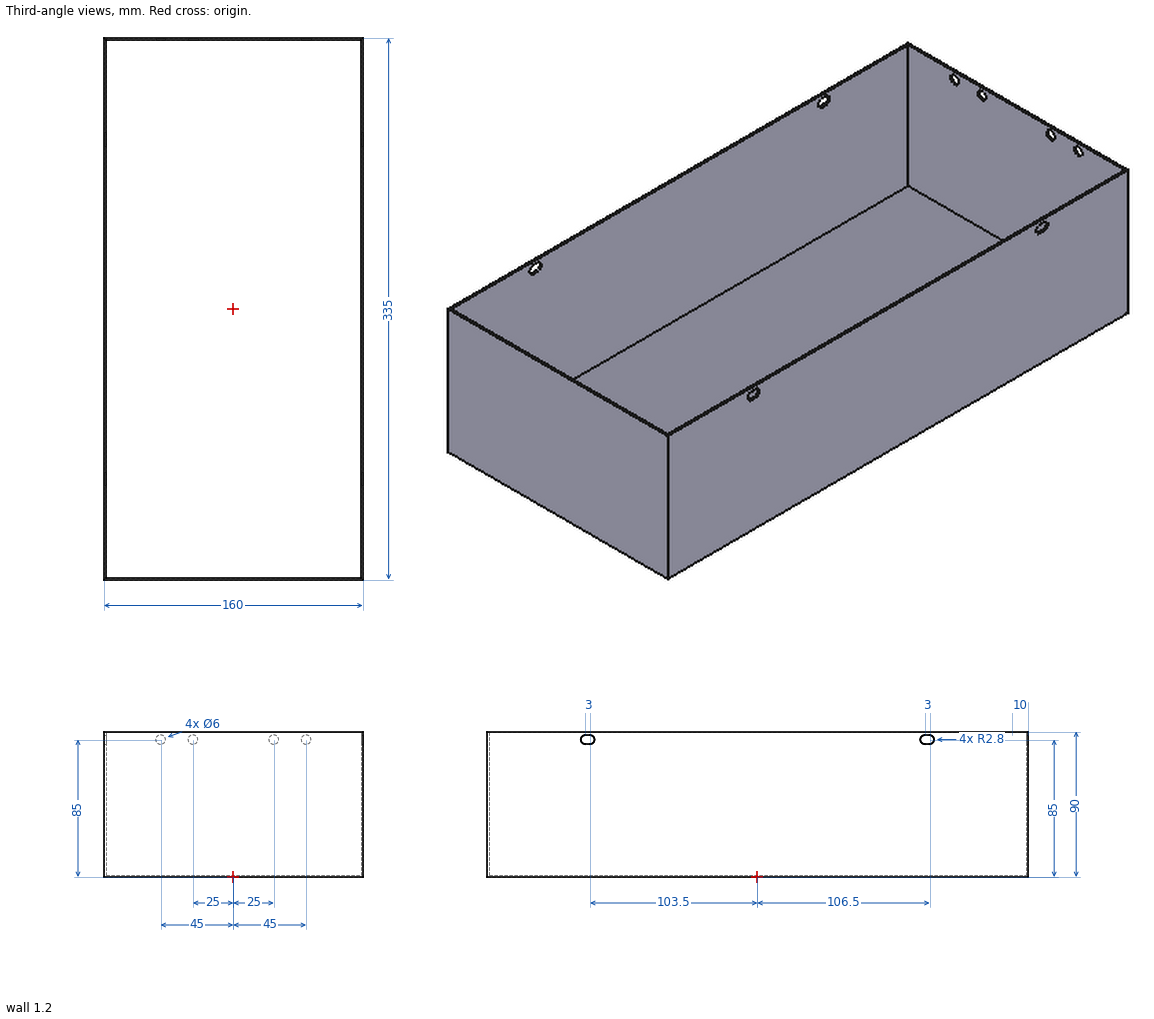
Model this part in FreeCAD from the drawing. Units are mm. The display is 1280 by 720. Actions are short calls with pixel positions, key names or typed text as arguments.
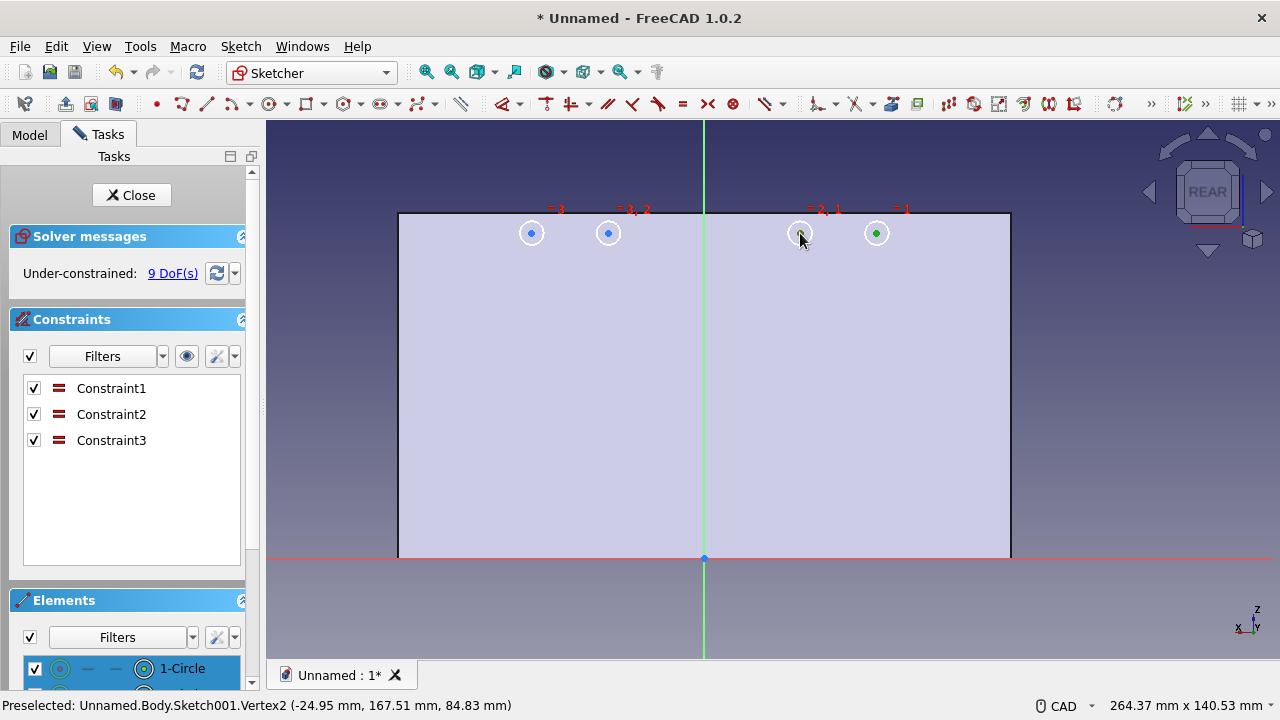
key(h)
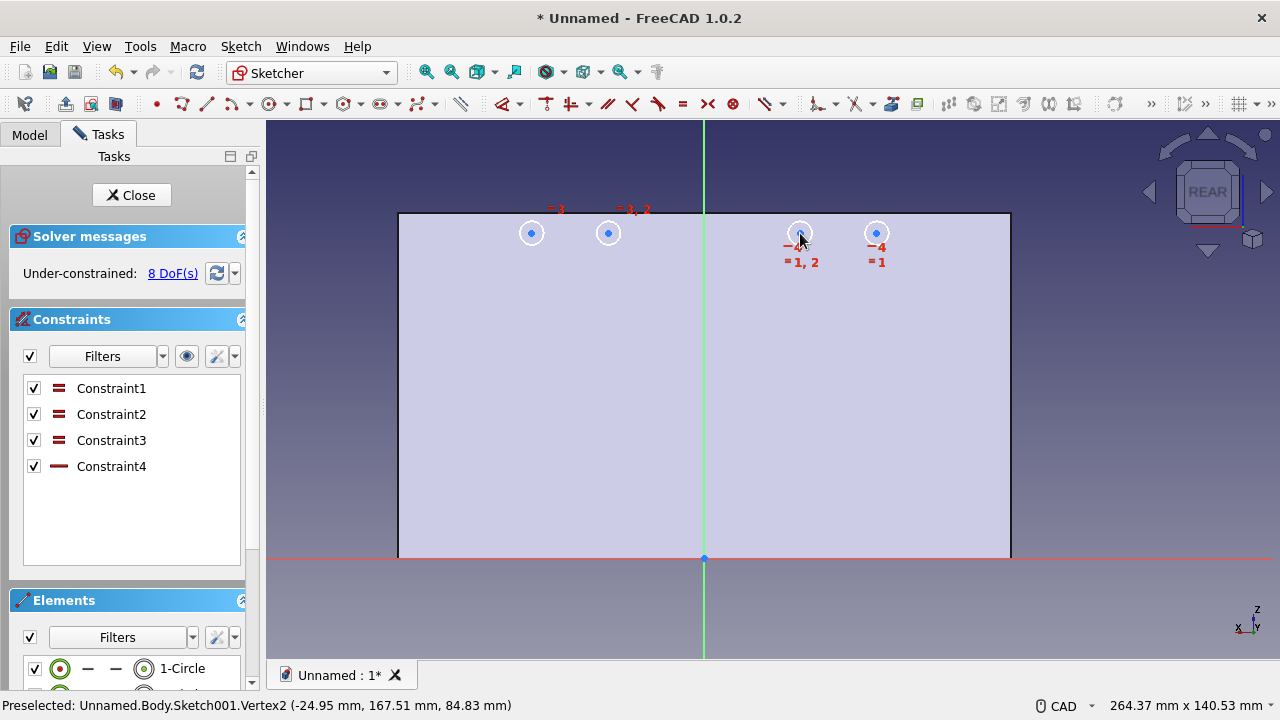
click(800, 233)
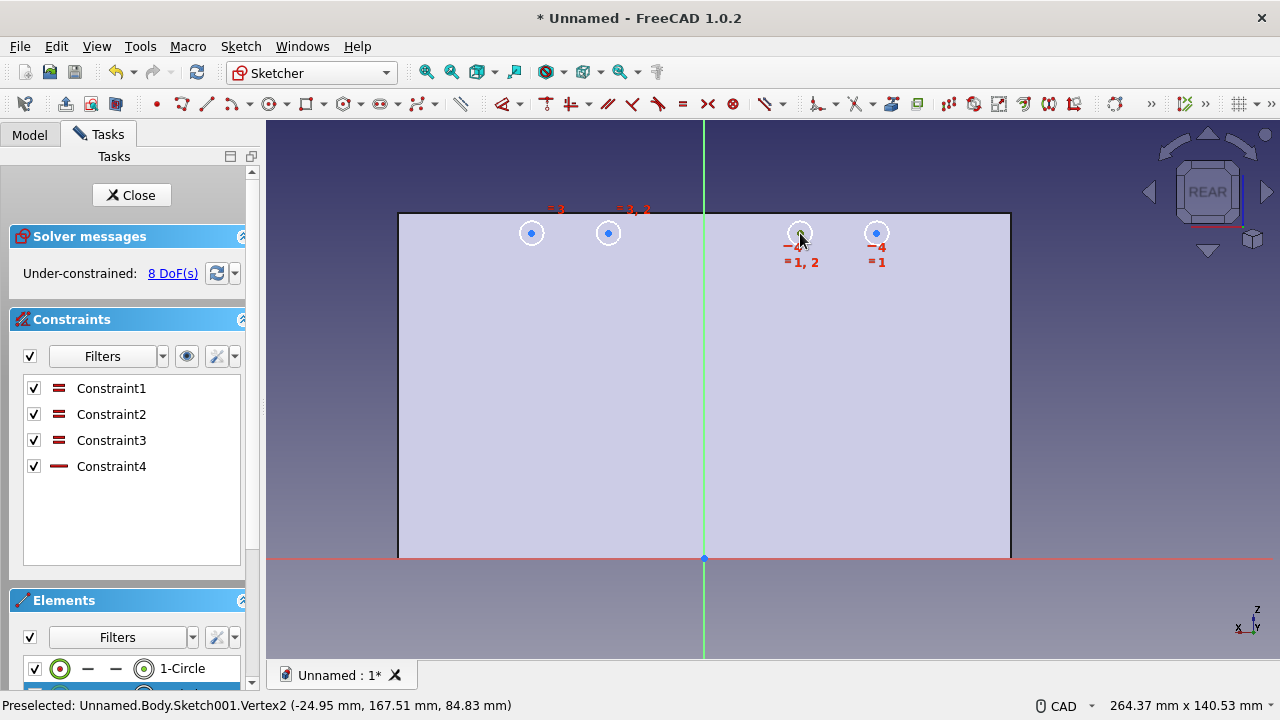
click(609, 233)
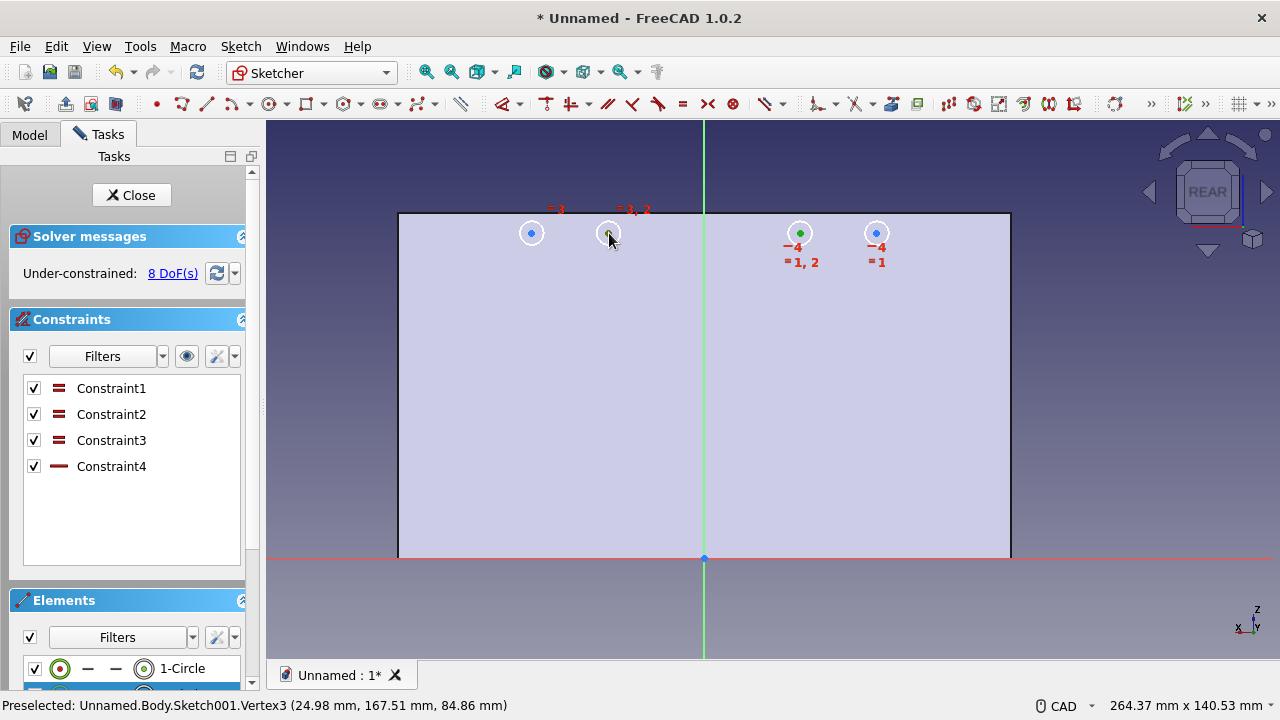
click(588, 104)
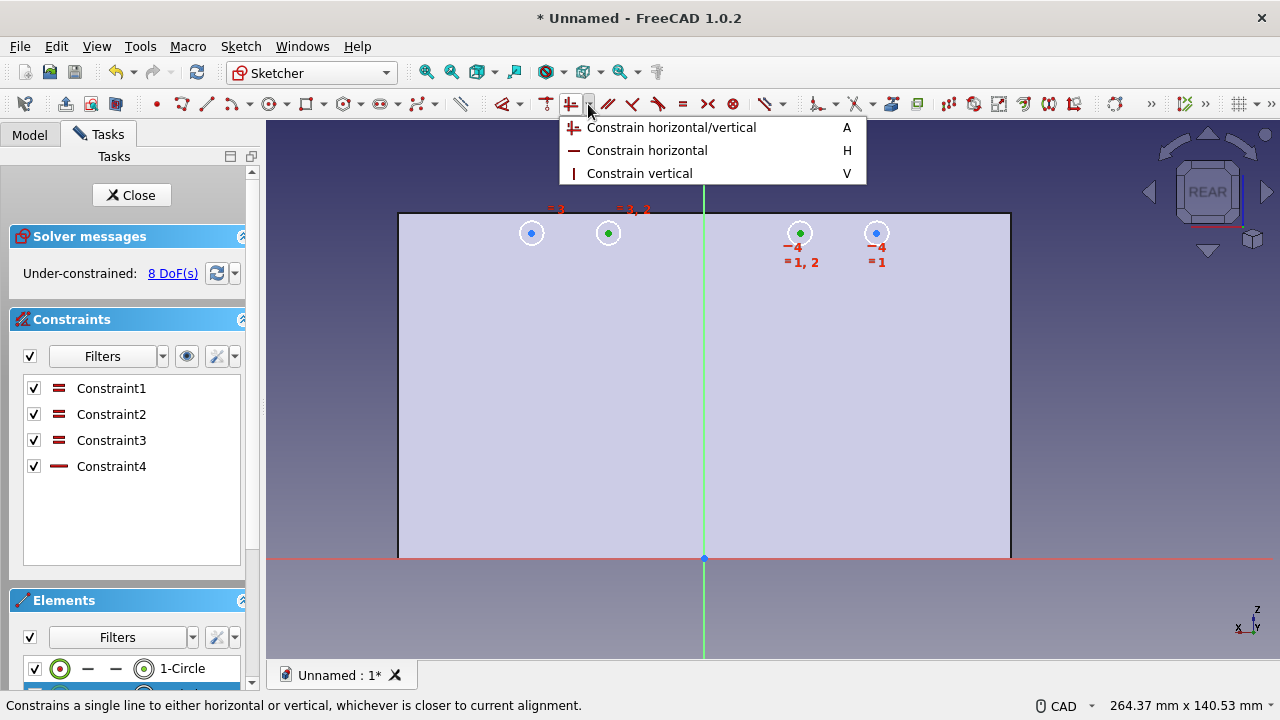
click(713, 150)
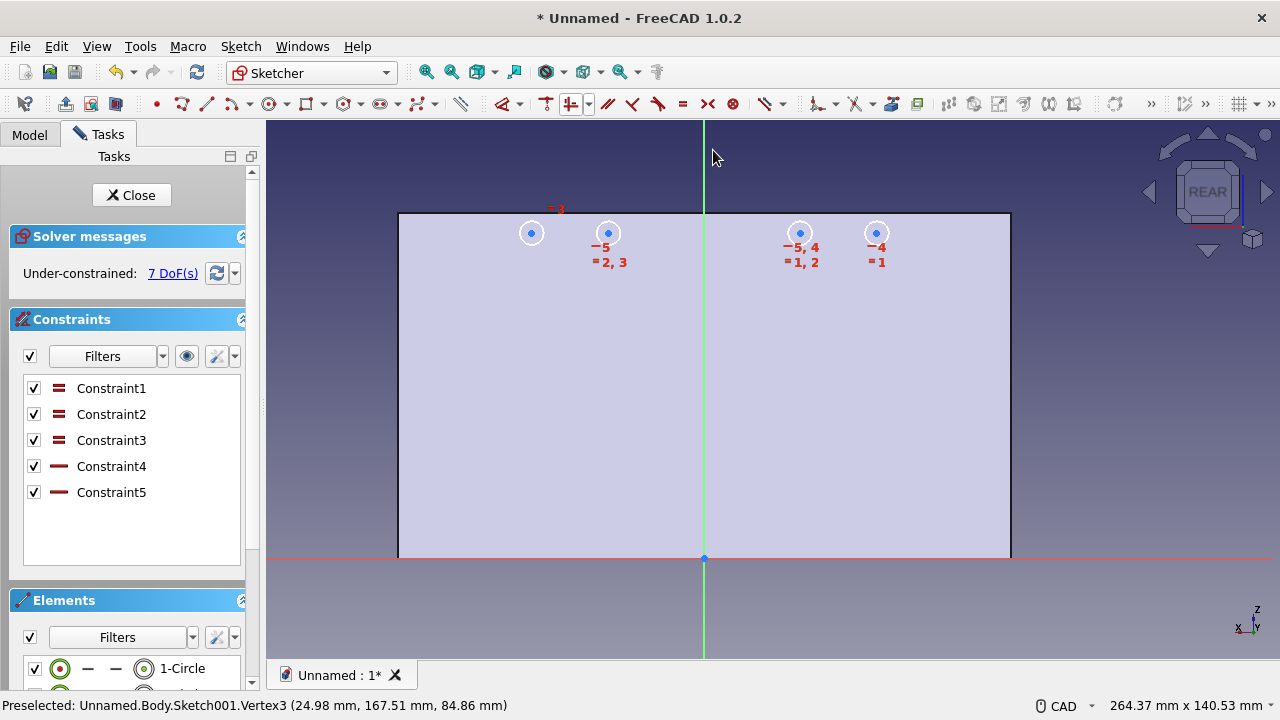
click(609, 233)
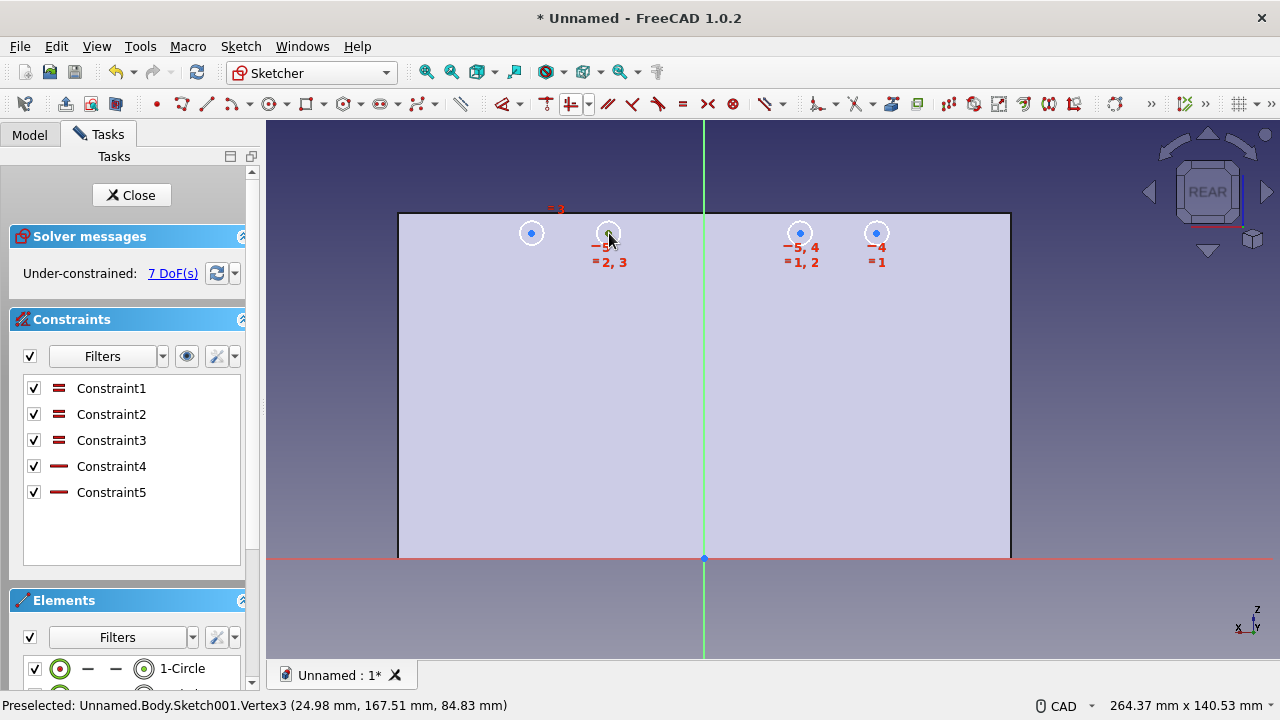
click(532, 233)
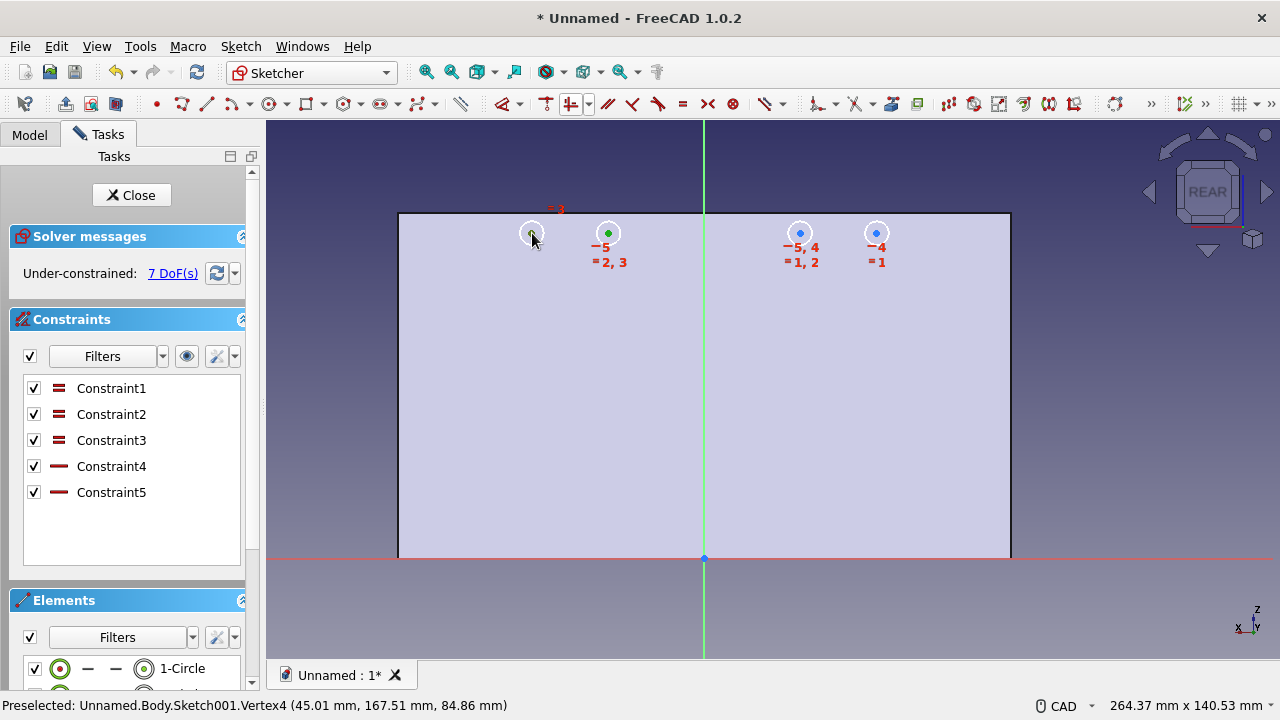
click(588, 104)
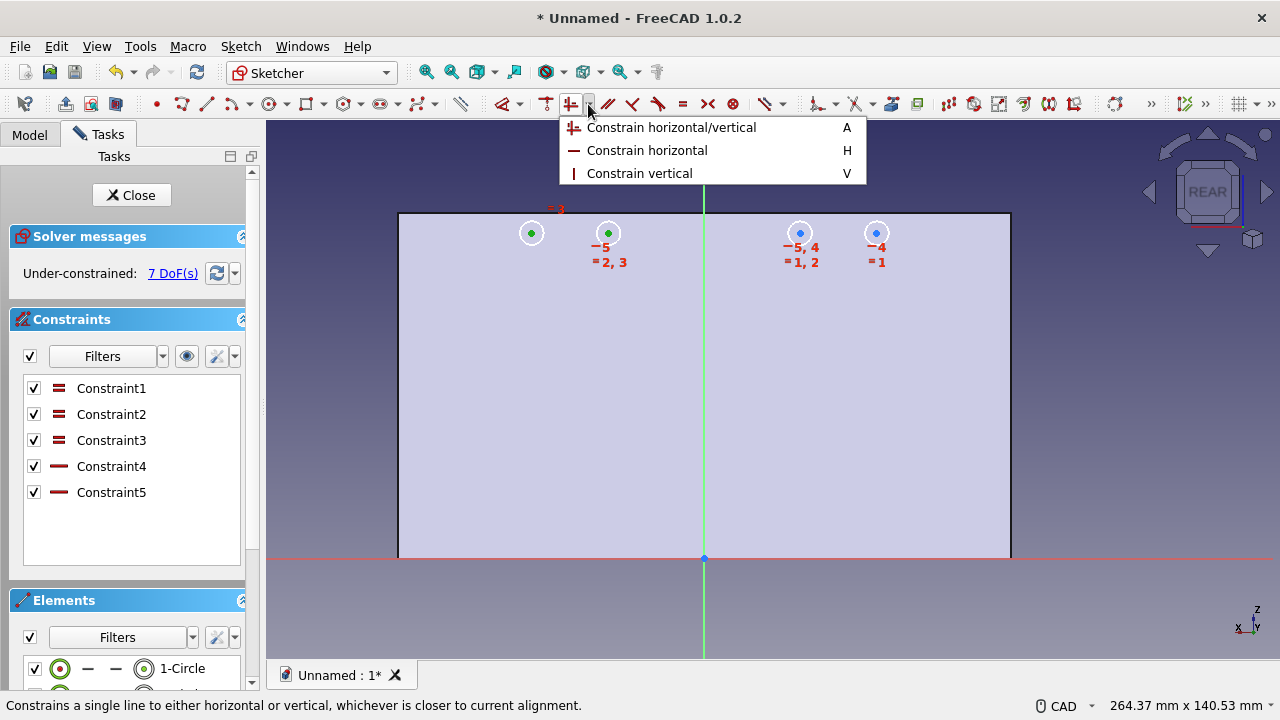
click(713, 150)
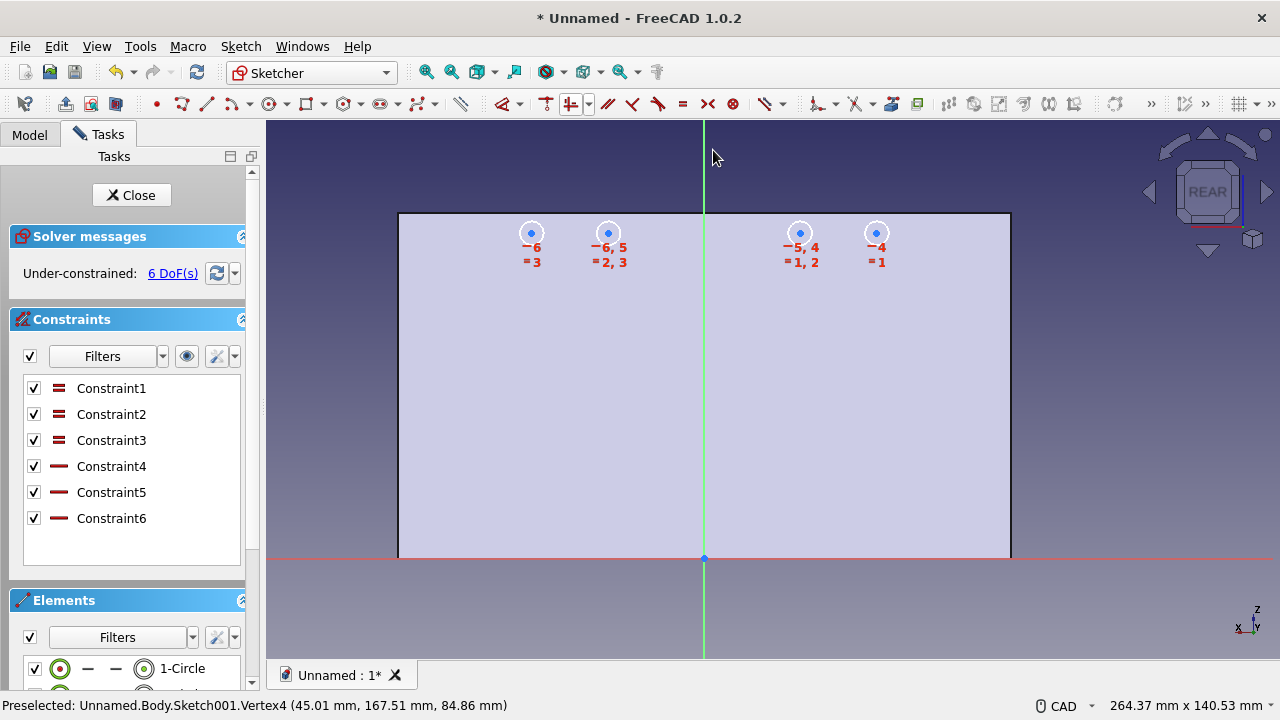
click(502, 104)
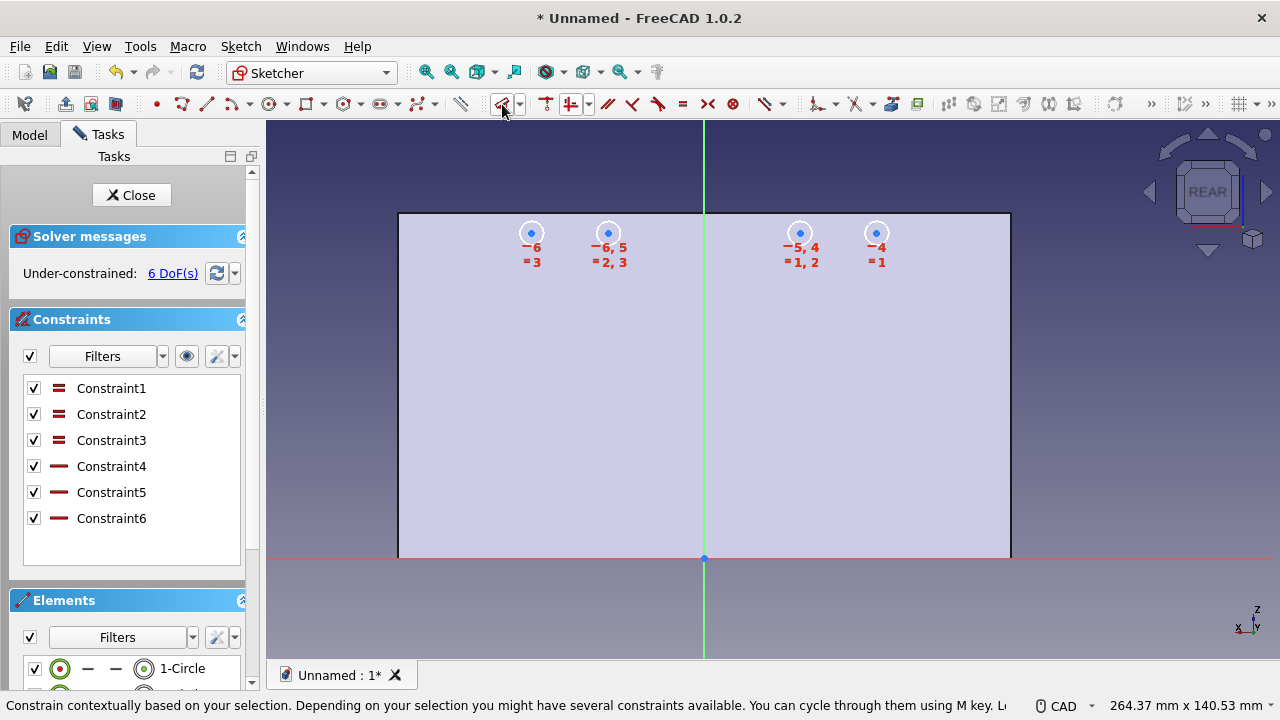
scroll(885, 225, up, 3)